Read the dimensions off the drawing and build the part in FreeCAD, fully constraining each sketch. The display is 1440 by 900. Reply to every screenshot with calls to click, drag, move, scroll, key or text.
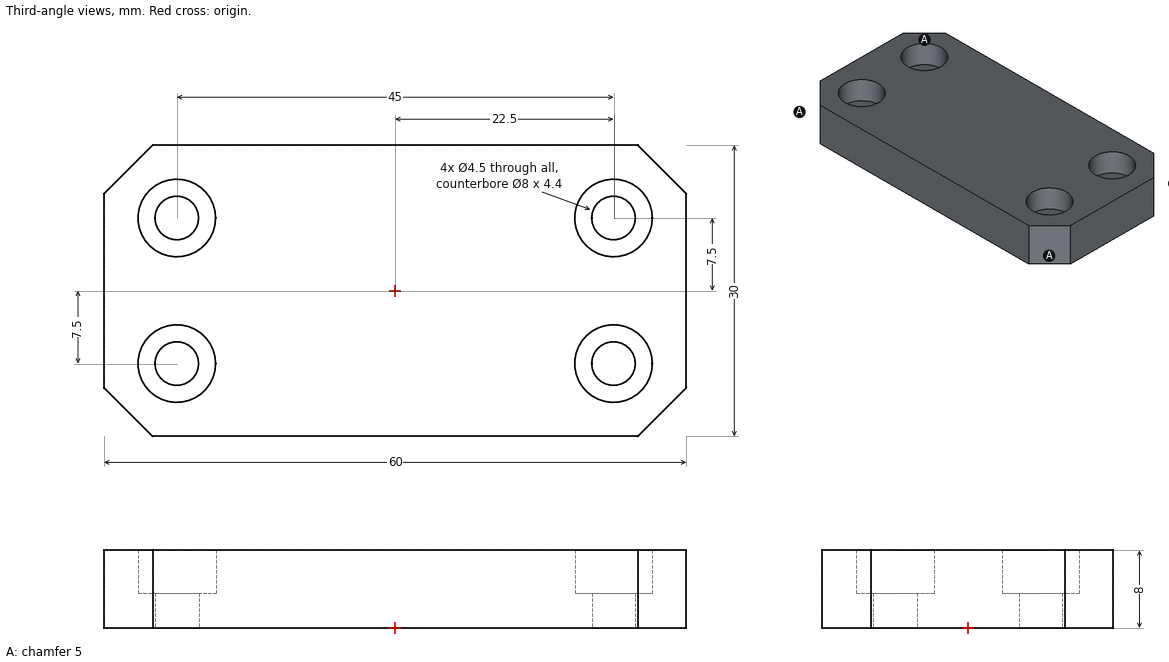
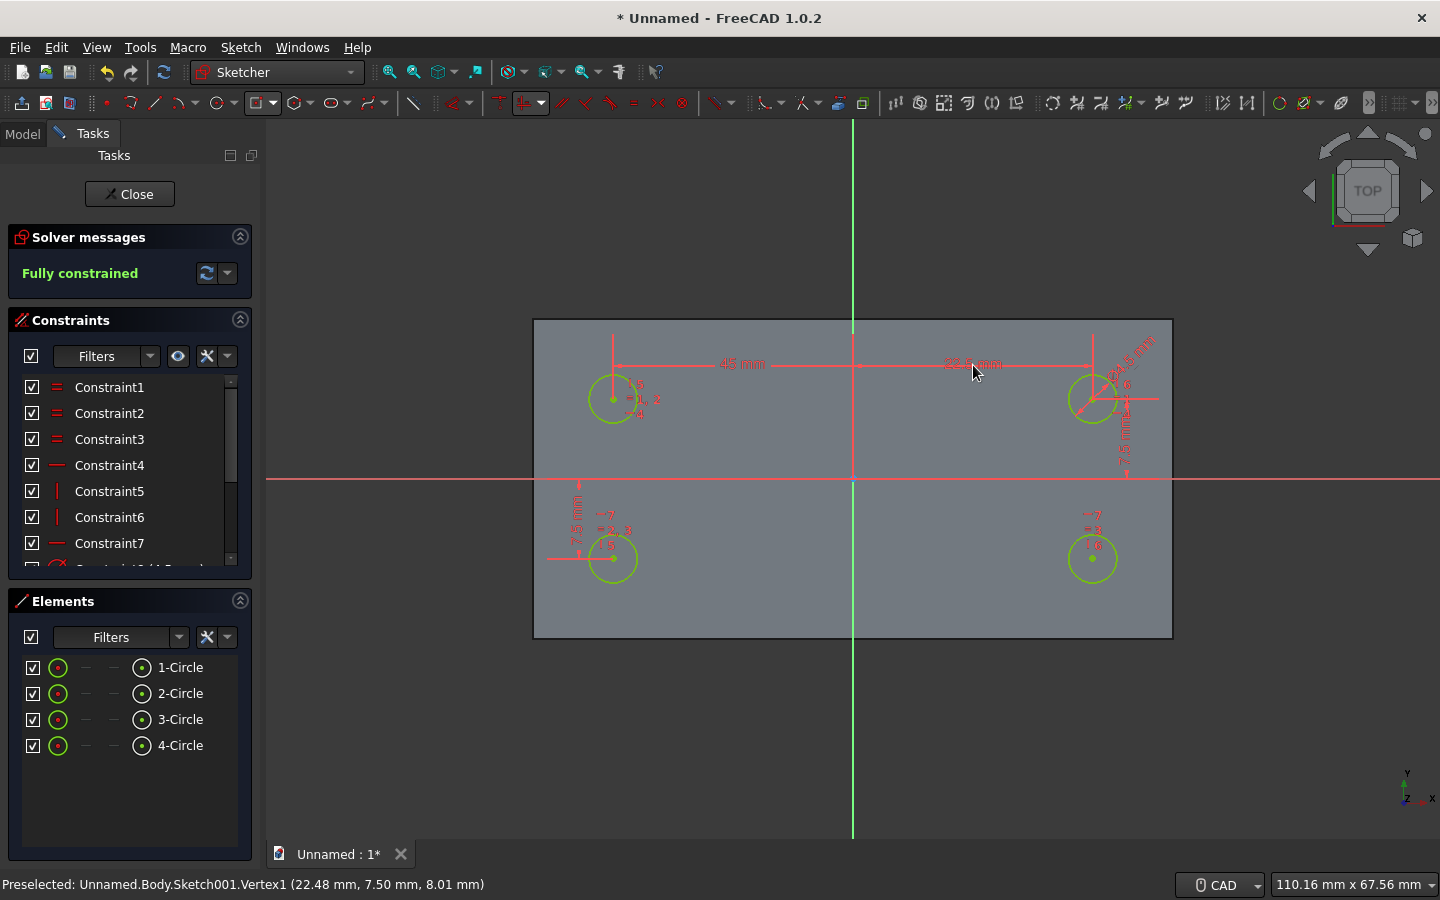
click(130, 194)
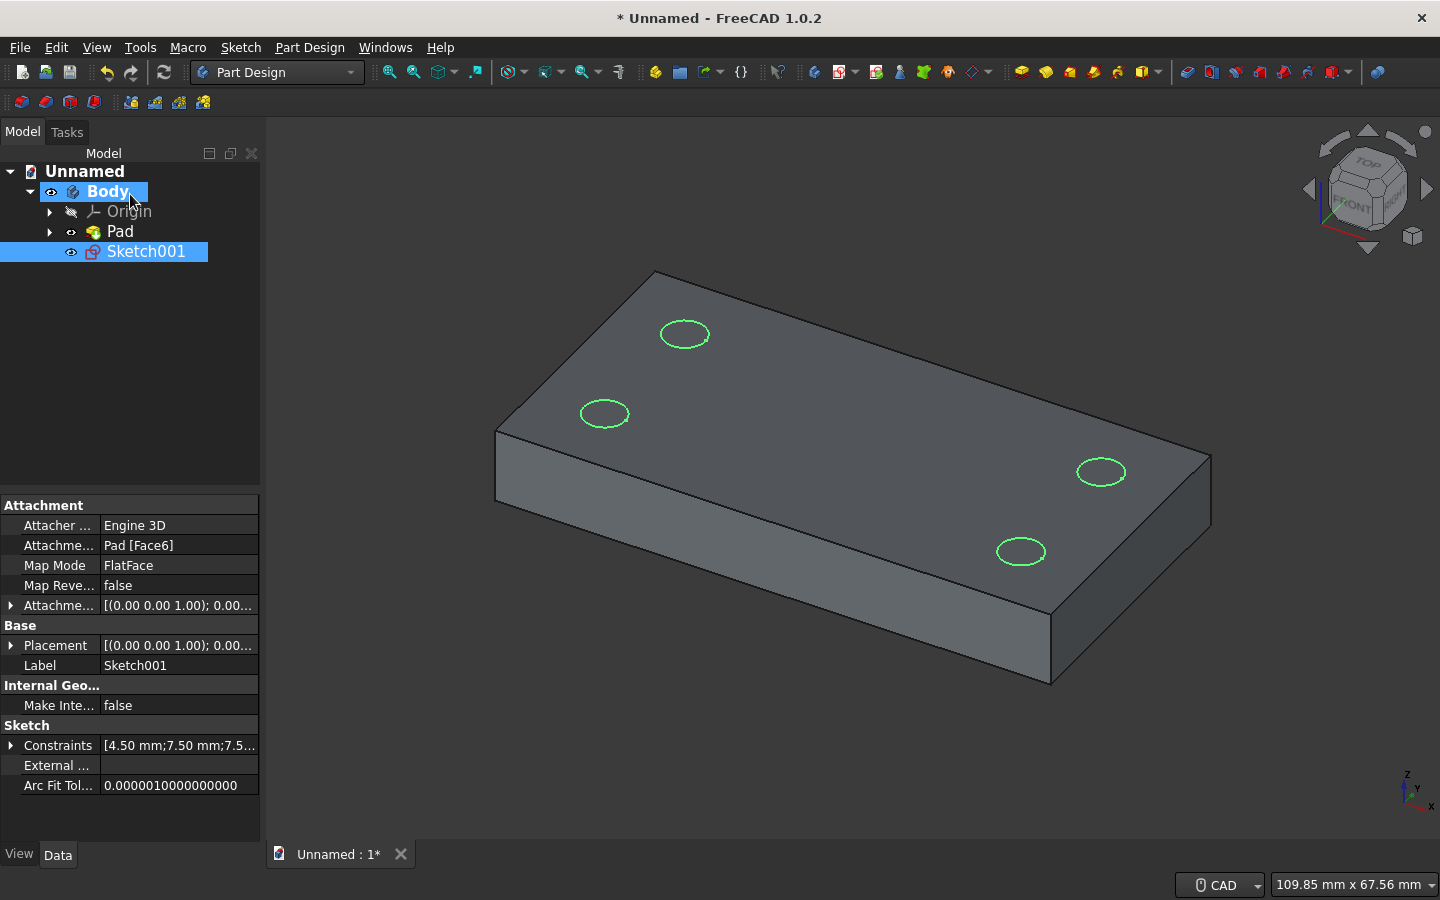
click(1212, 72)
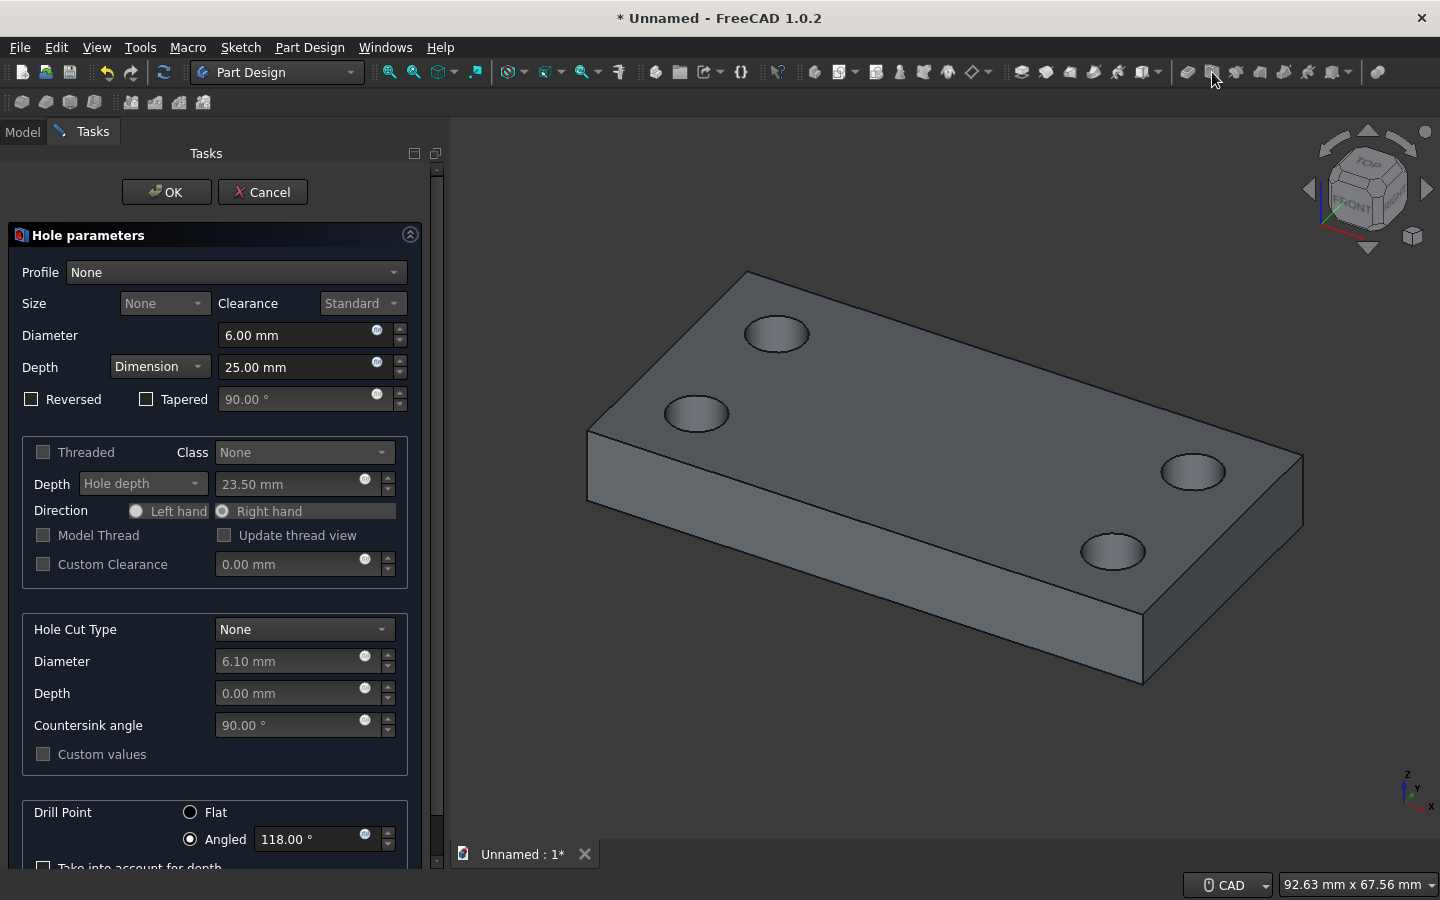
triple_click(305, 335)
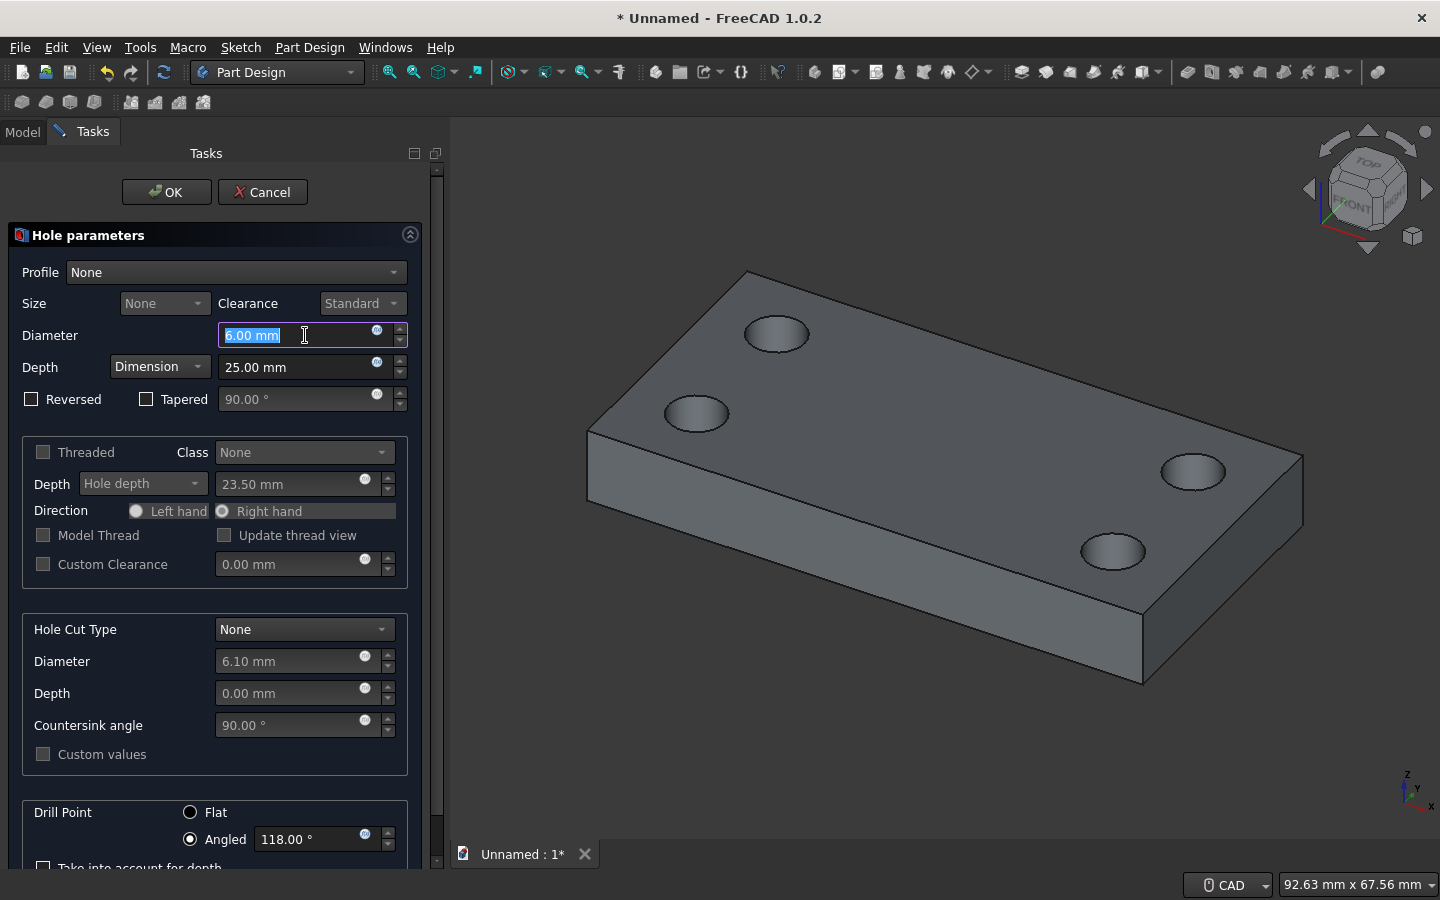
text(4.5)
key(Tab)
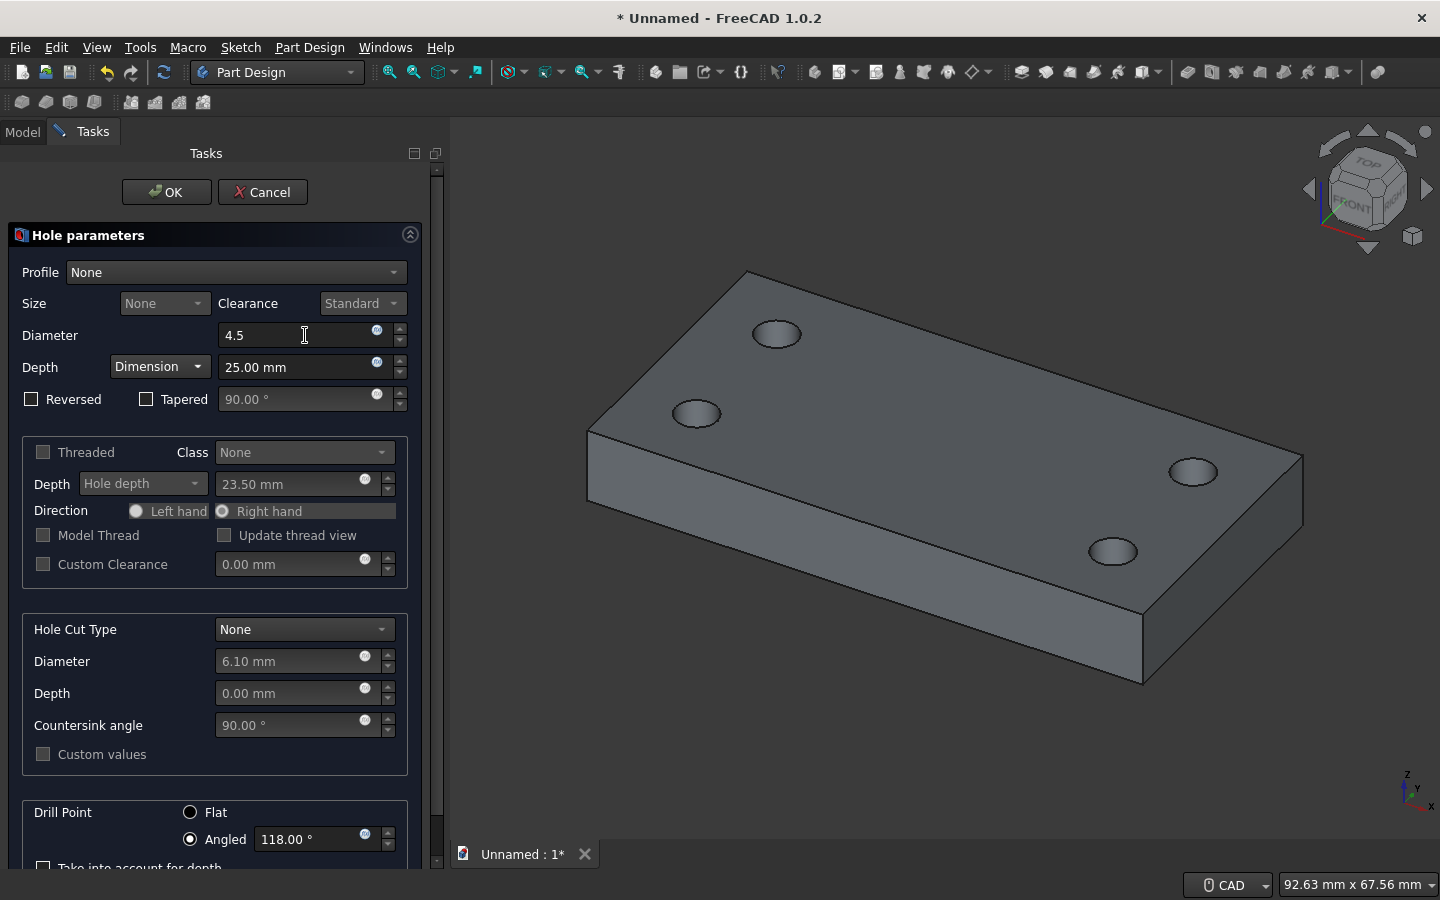
click(161, 366)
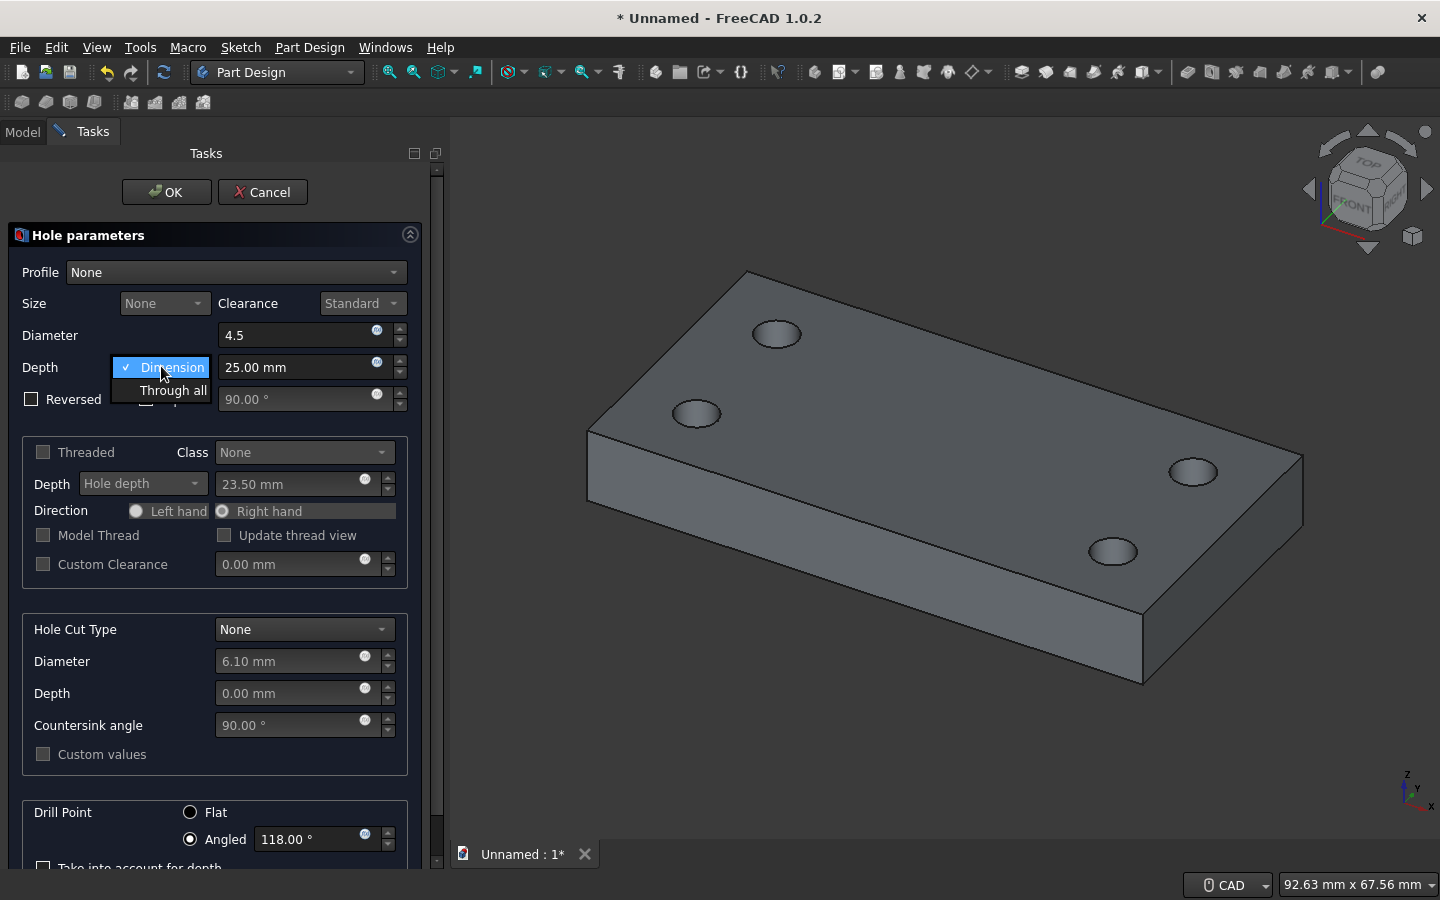
click(160, 390)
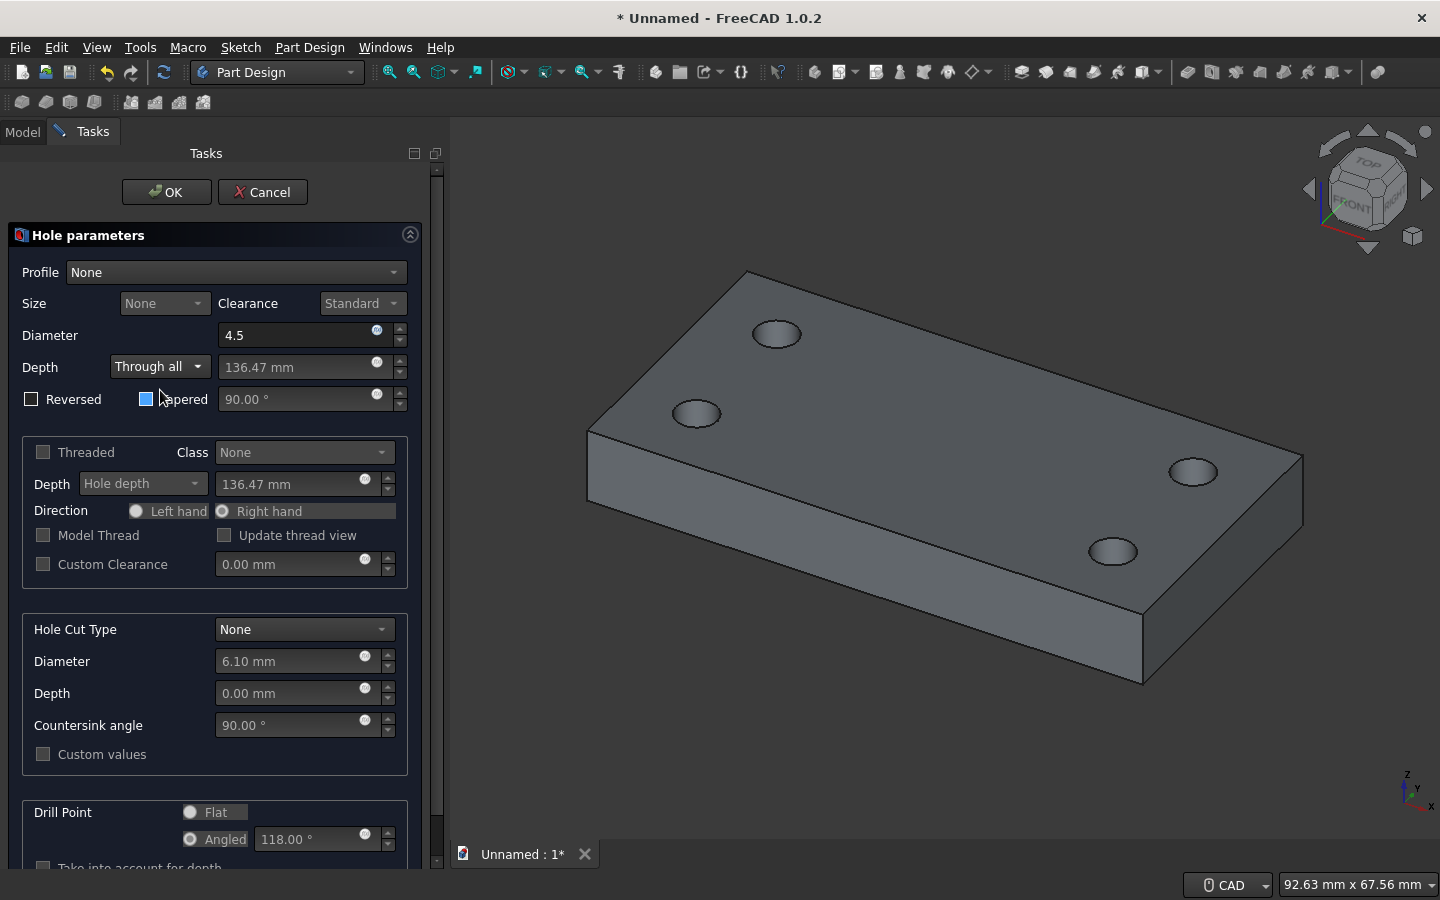
click(306, 630)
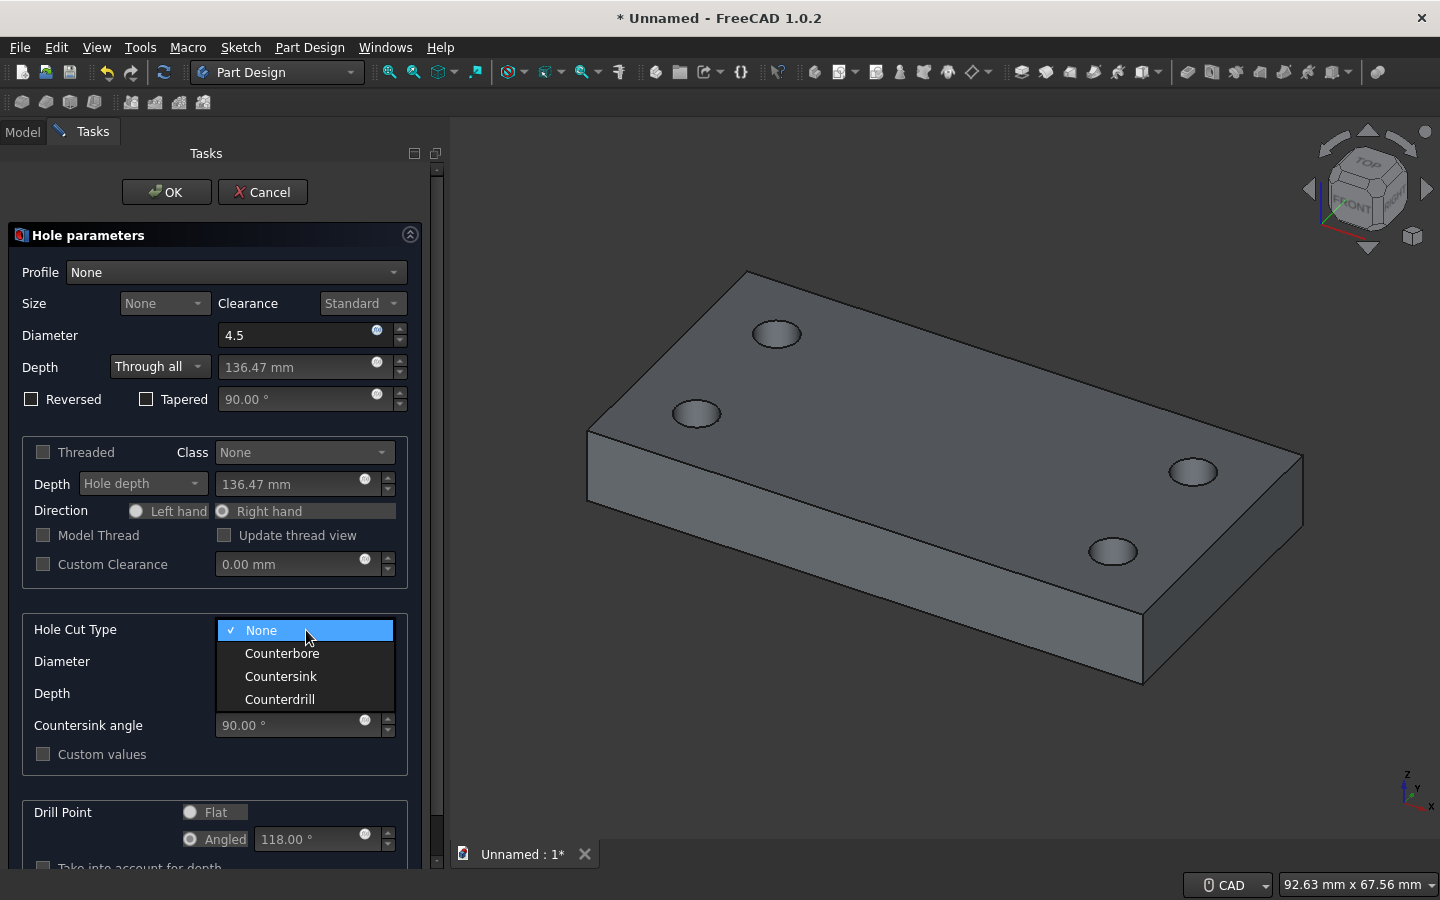
click(304, 654)